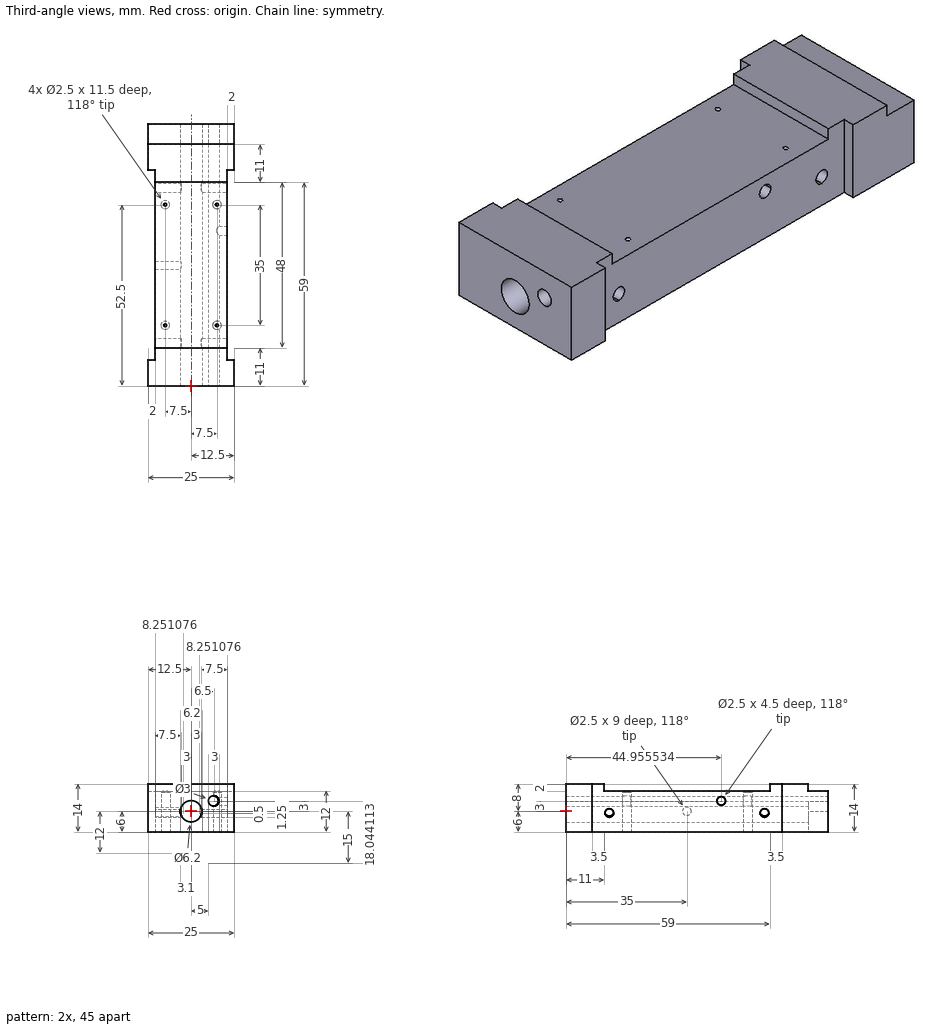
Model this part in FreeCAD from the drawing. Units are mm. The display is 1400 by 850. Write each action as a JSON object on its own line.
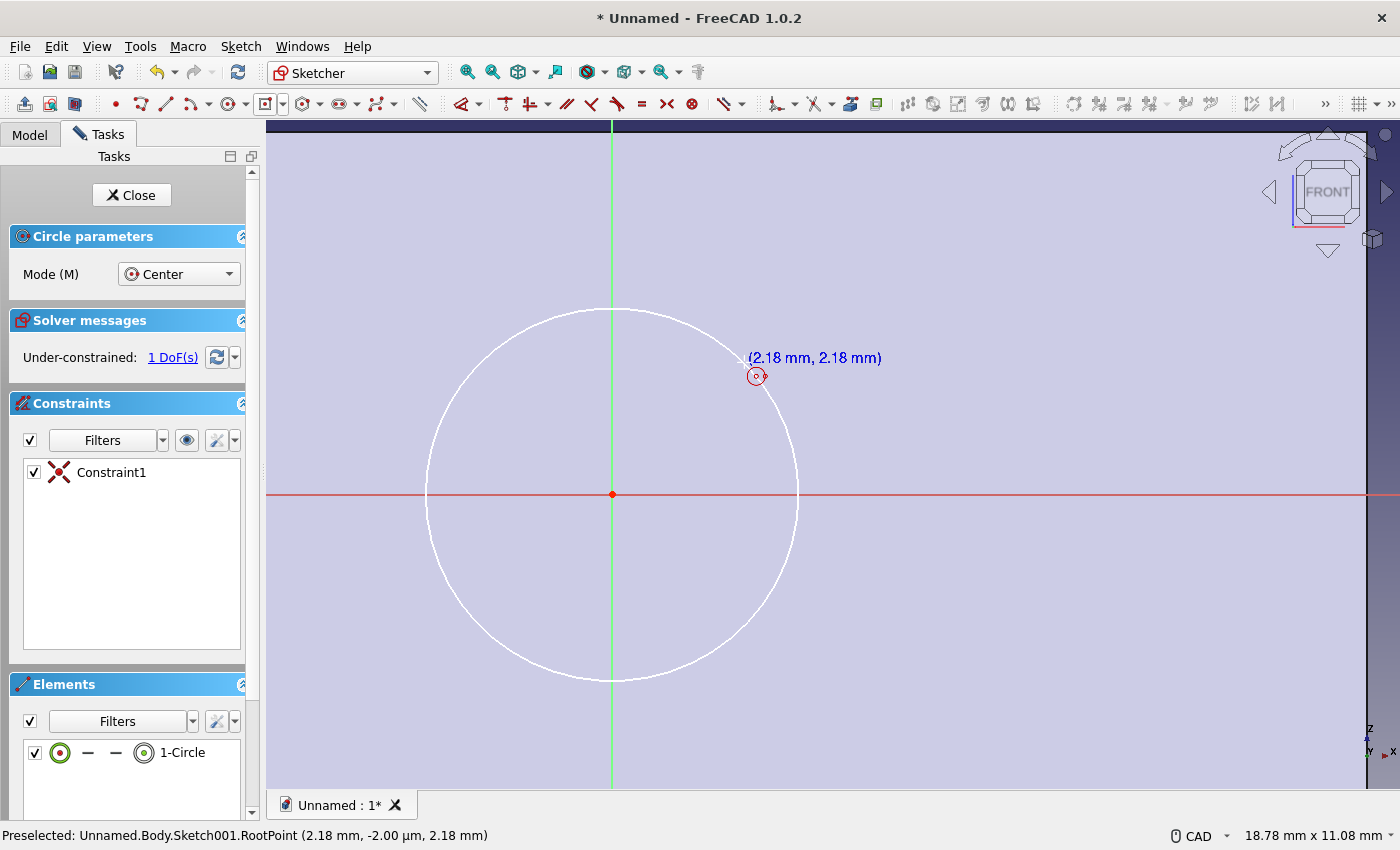
{"action": "left_click", "coordinate": [1005, 314]}
{"action": "left_click", "coordinate": [1069, 250]}
{"action": "key", "text": "Escape"}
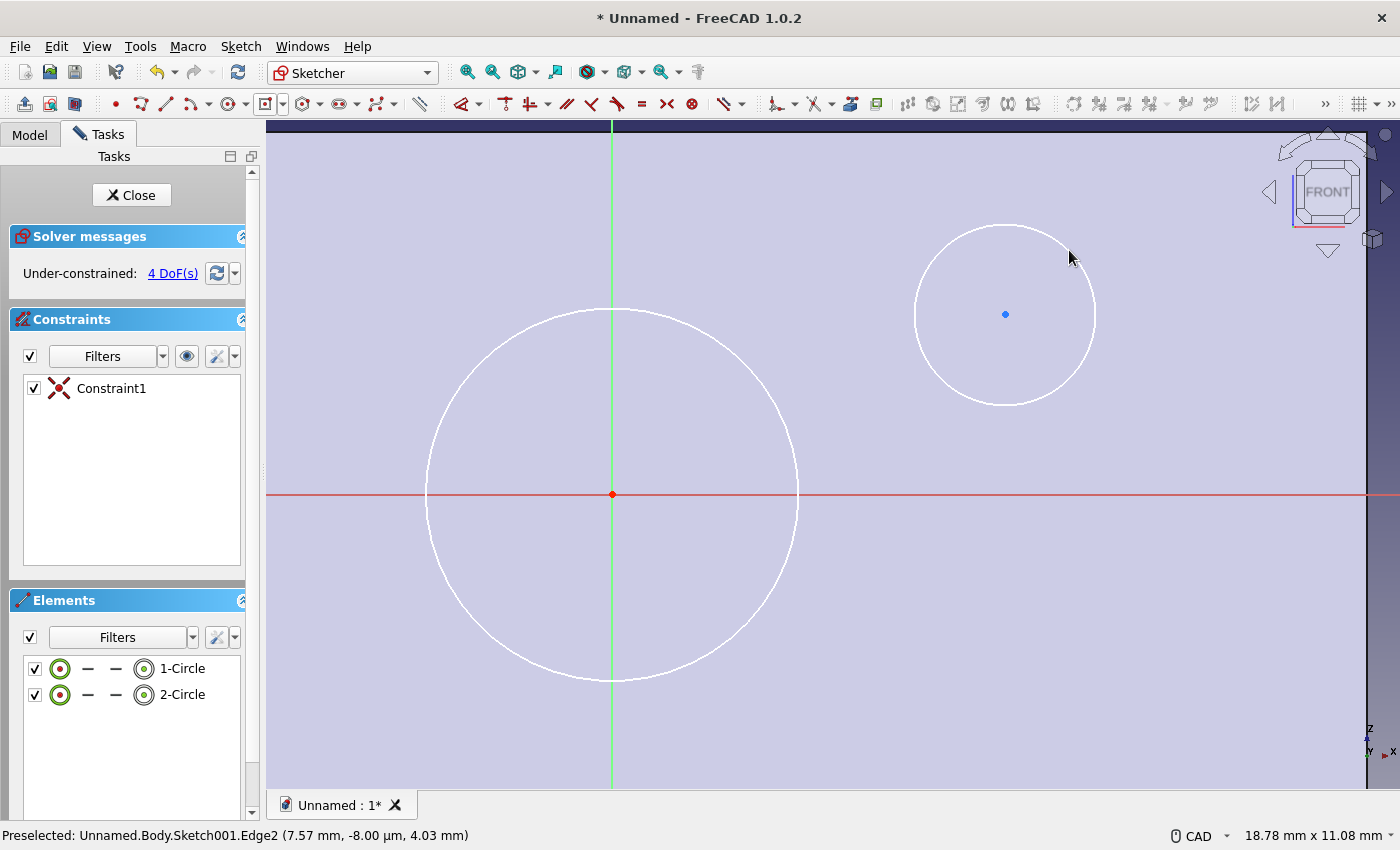
{"action": "left_click", "coordinate": [460, 104]}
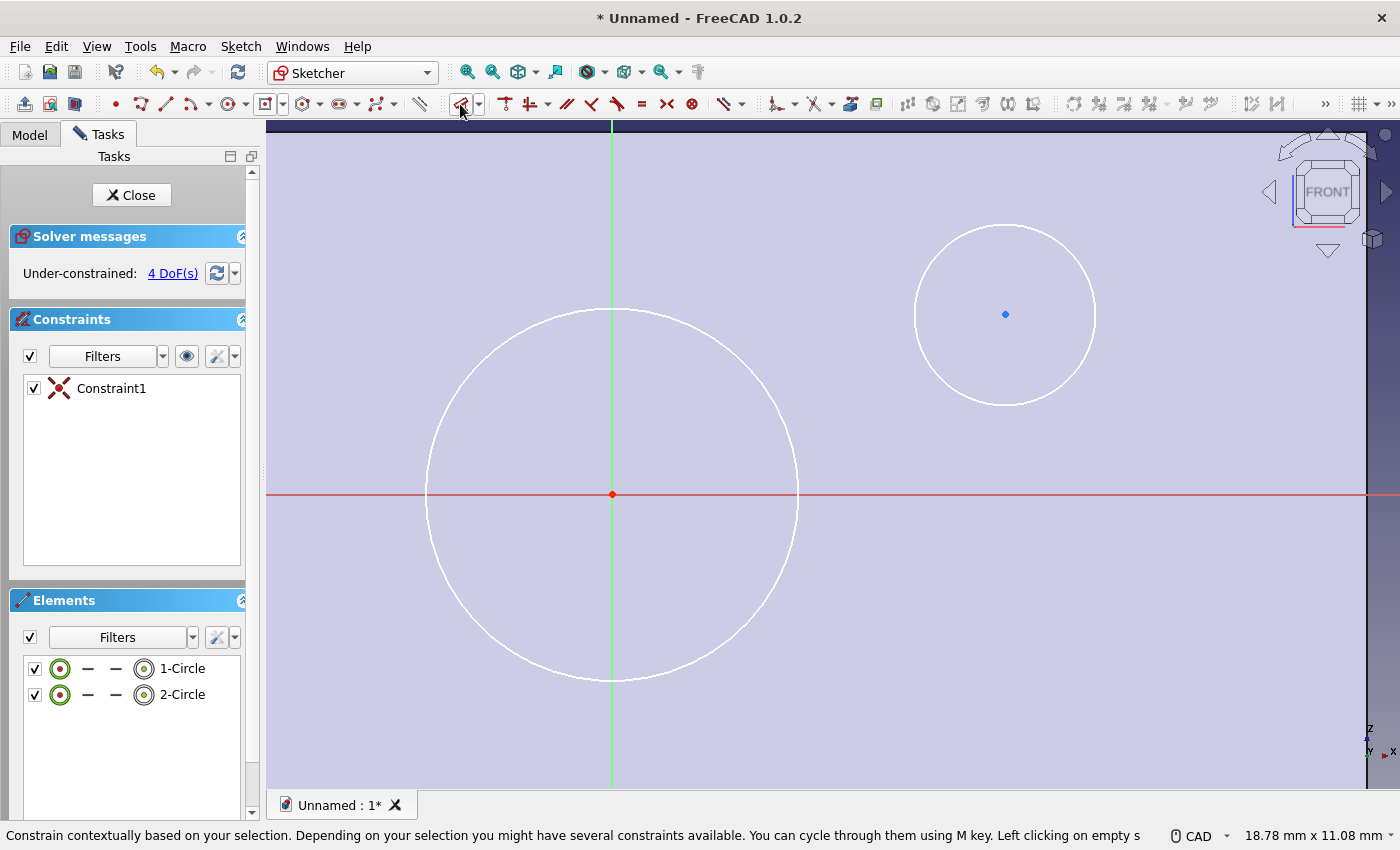
{"action": "left_click", "coordinate": [743, 362]}
{"action": "left_click", "coordinate": [765, 339]}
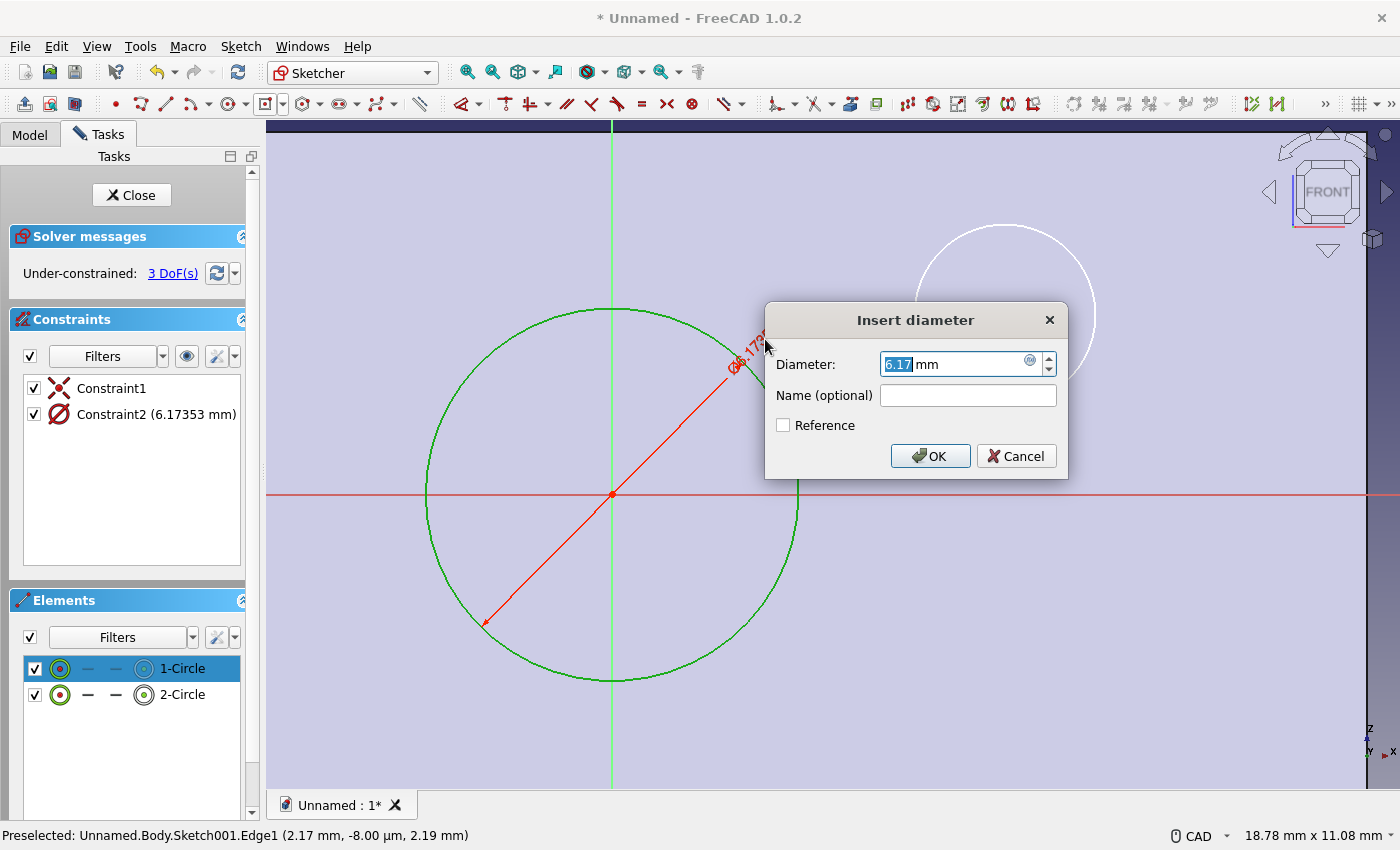
{"action": "type", "text": "6.2"}
{"action": "key", "text": "Return"}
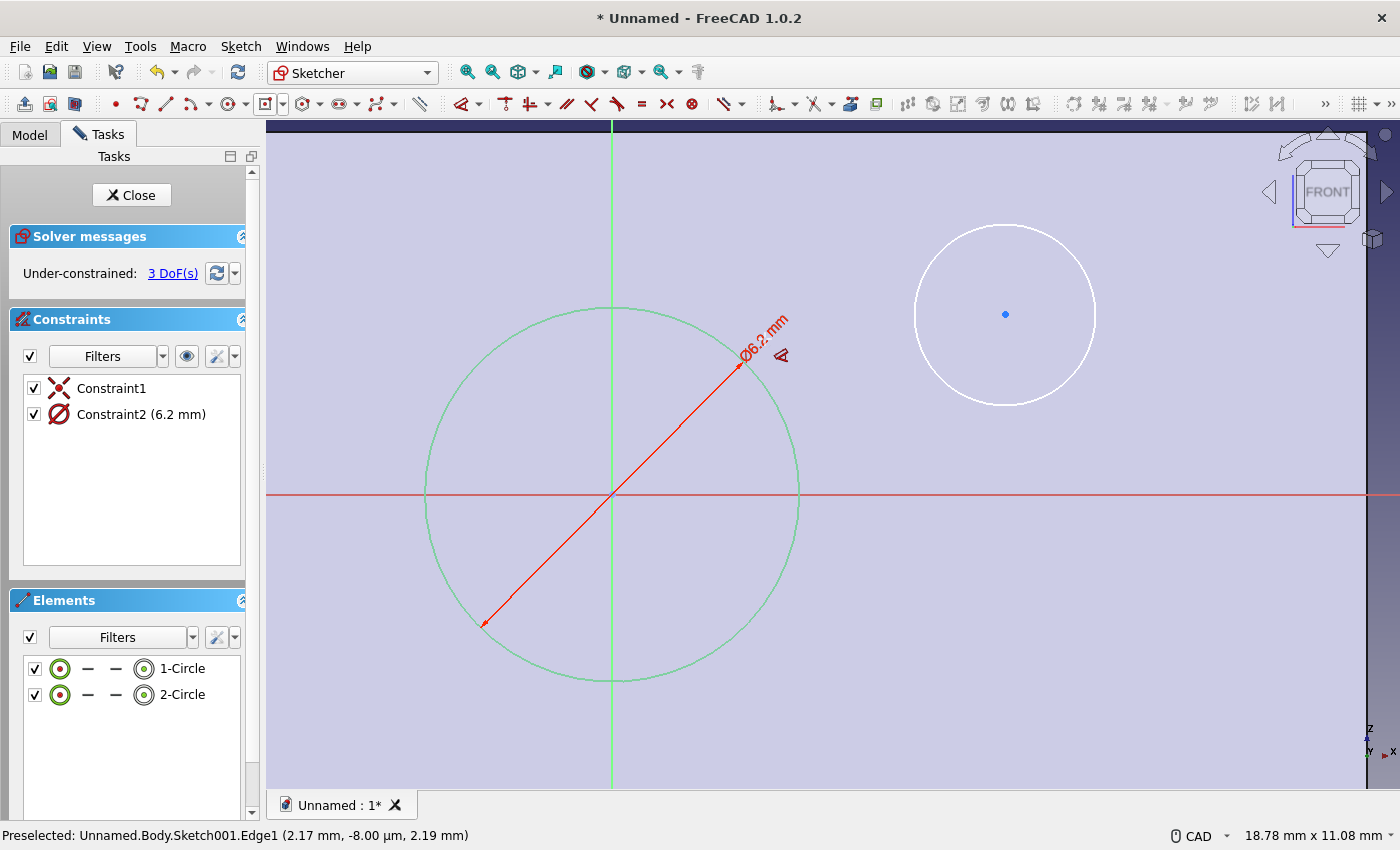
{"action": "left_click", "coordinate": [1069, 251]}
{"action": "left_click", "coordinate": [1092, 228]}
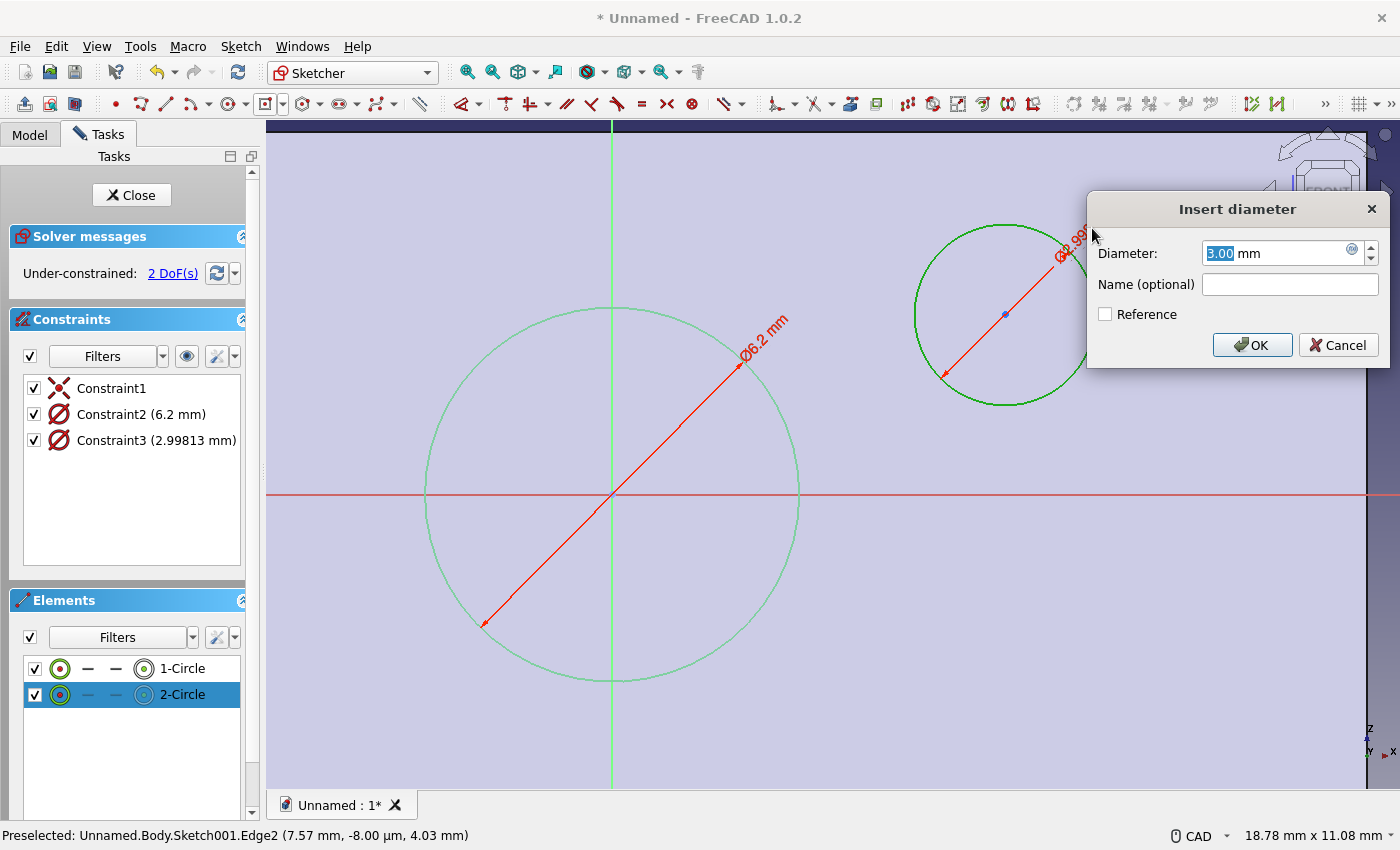
{"action": "type", "text": "3"}
{"action": "key", "text": "Return"}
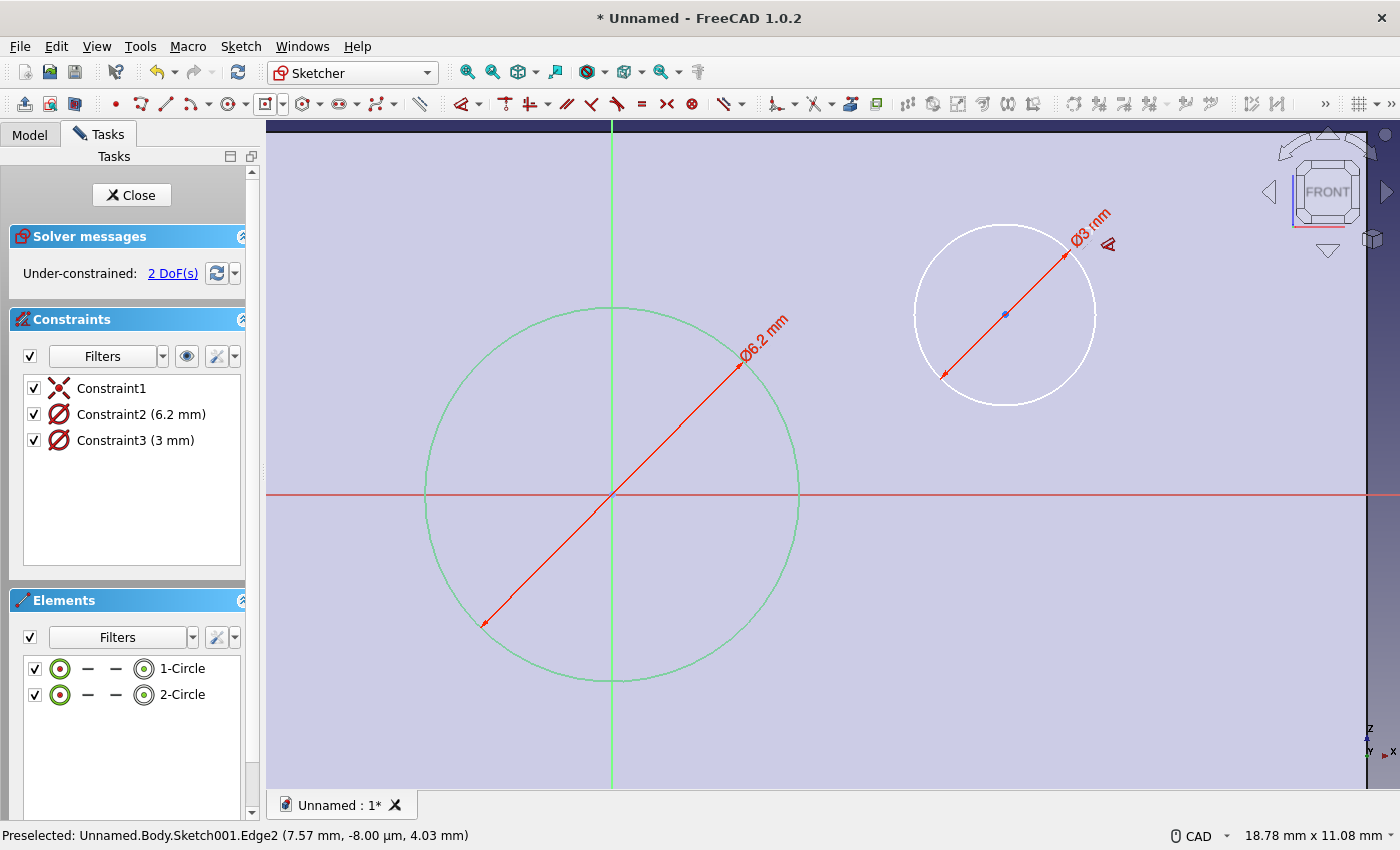
{"action": "left_click", "coordinate": [1005, 315]}
{"action": "left_click", "coordinate": [1039, 364]}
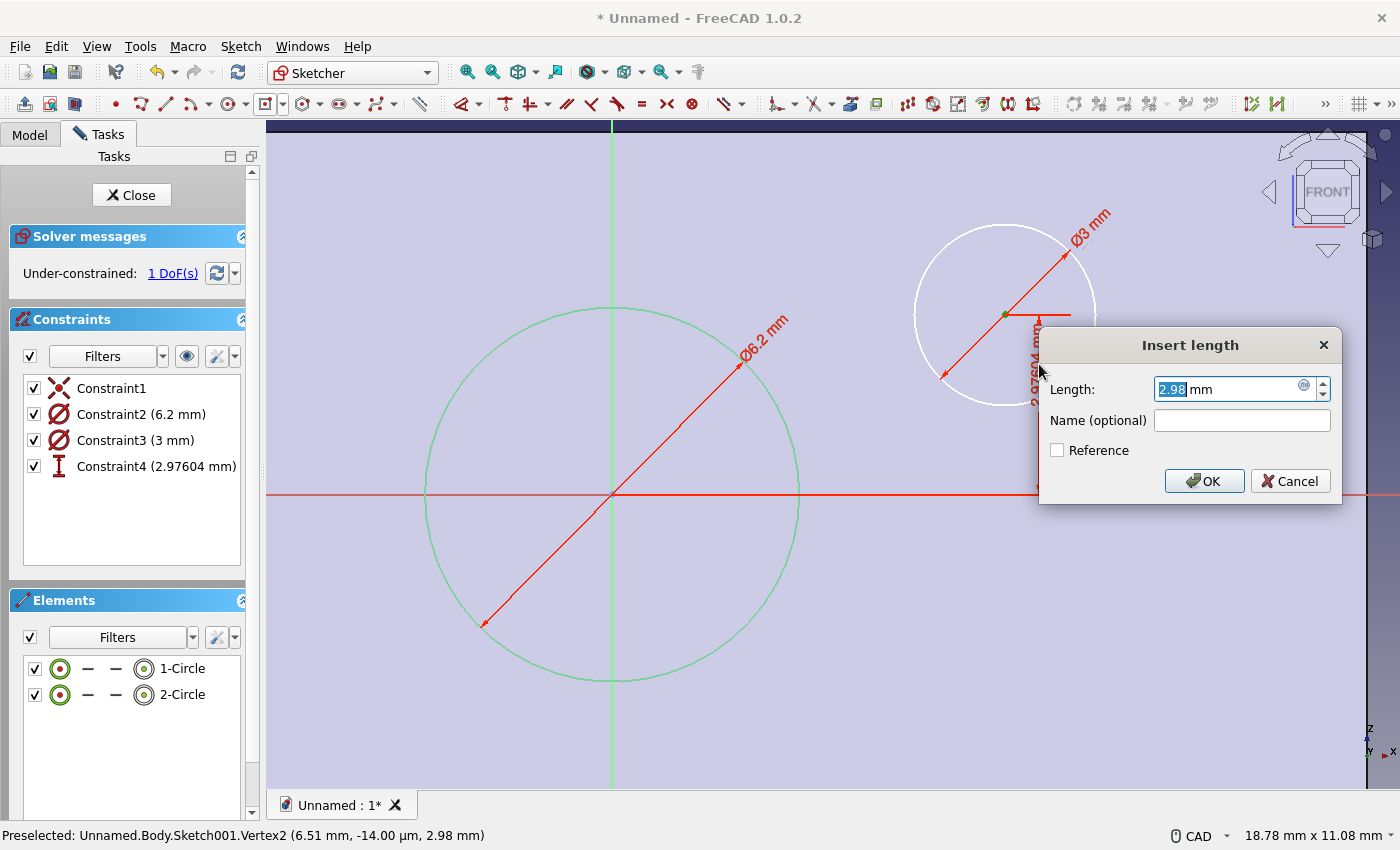
{"action": "type", "text": "3"}
{"action": "key", "text": "Return"}